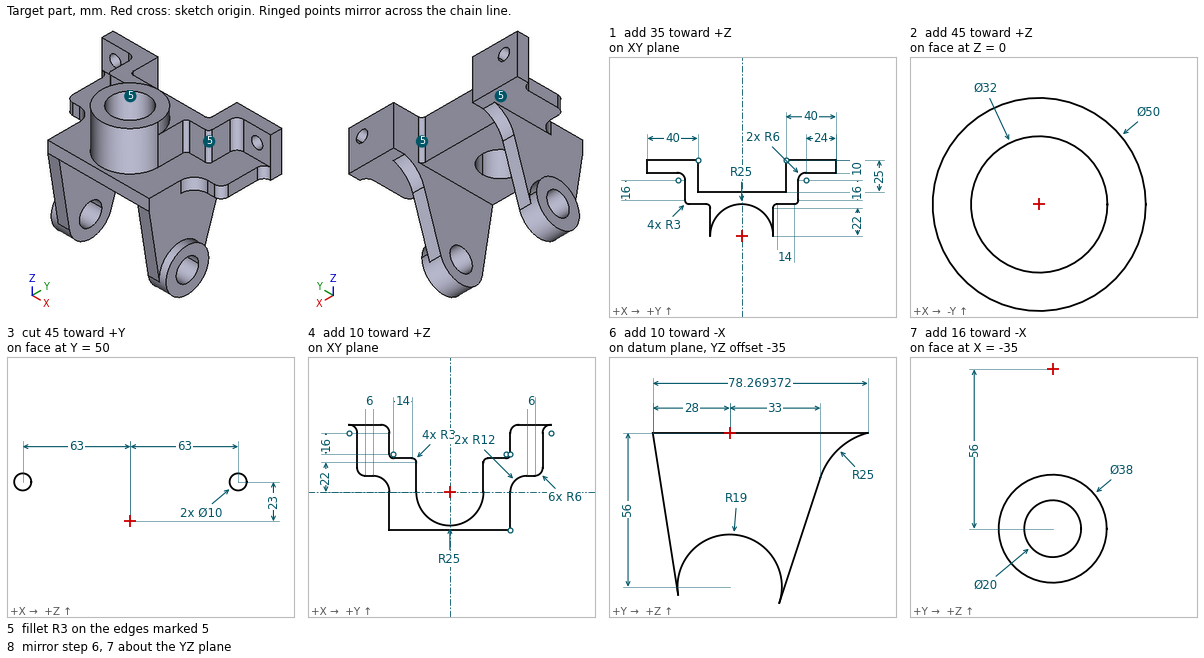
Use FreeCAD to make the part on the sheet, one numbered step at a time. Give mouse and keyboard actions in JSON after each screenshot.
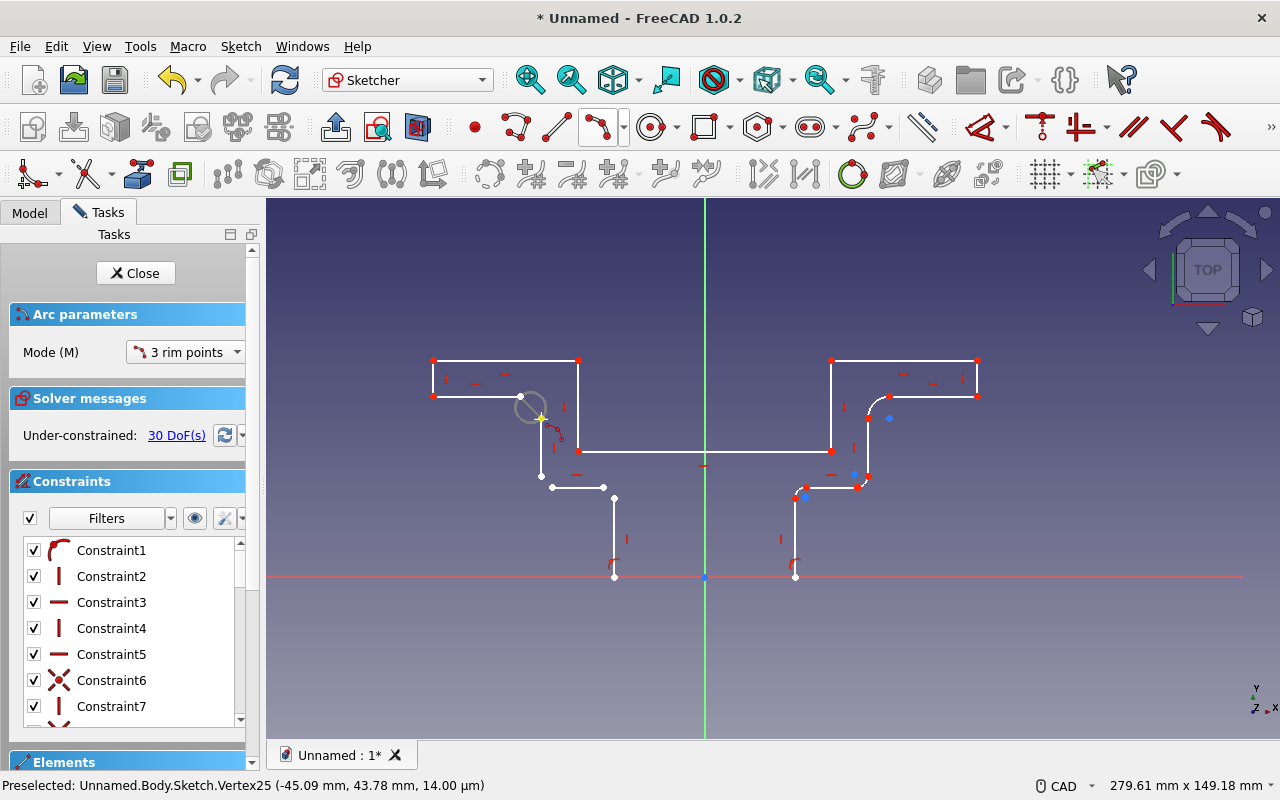
{"action": "scroll", "coordinate": [535, 402], "scroll_direction": "up", "scroll_amount": 5}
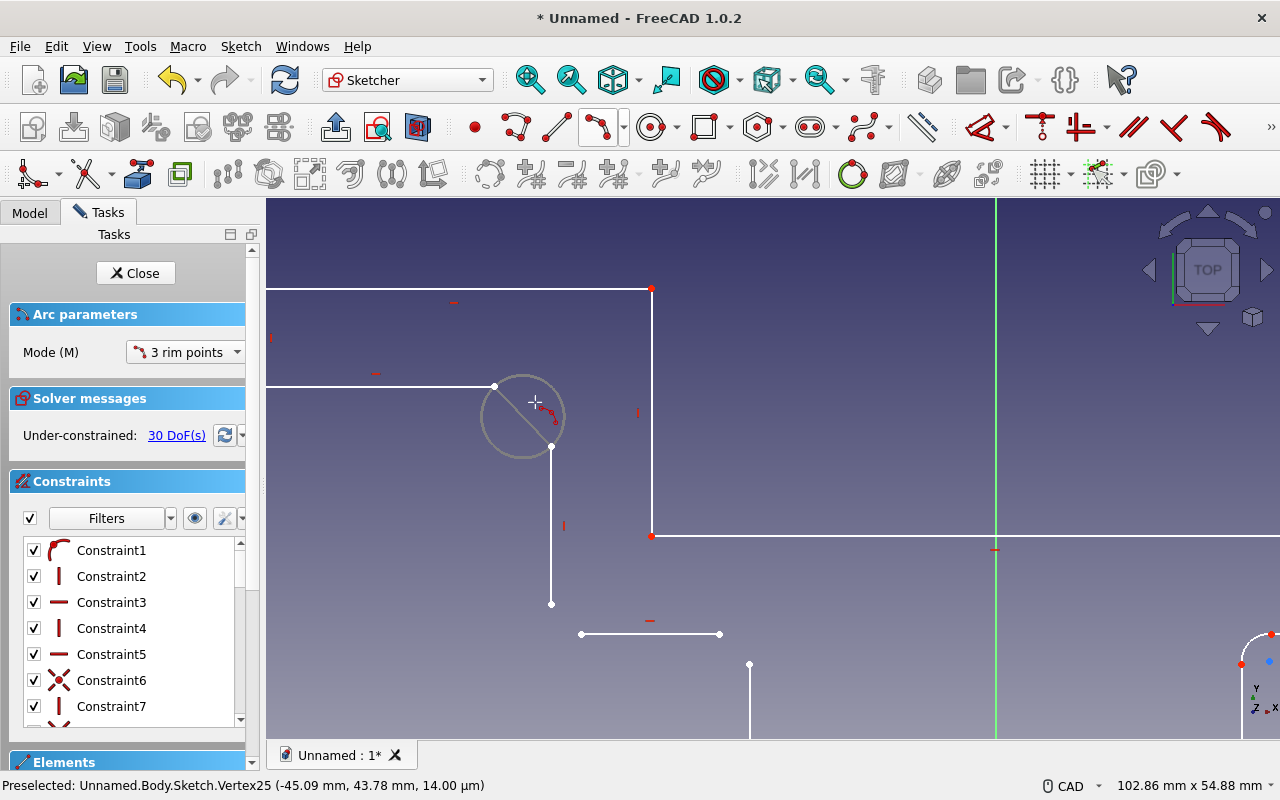
{"action": "left_click", "coordinate": [535, 403]}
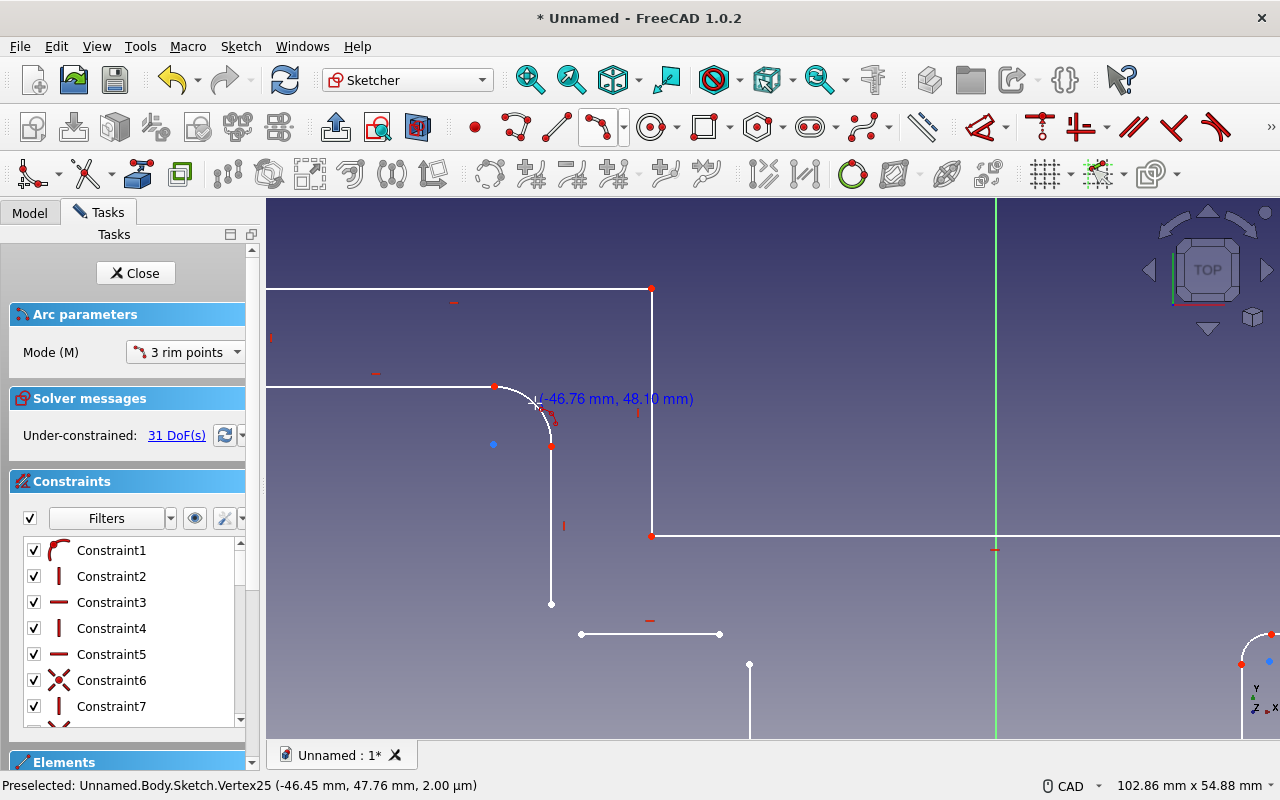
{"action": "left_click", "coordinate": [551, 604]}
{"action": "left_click", "coordinate": [581, 634]}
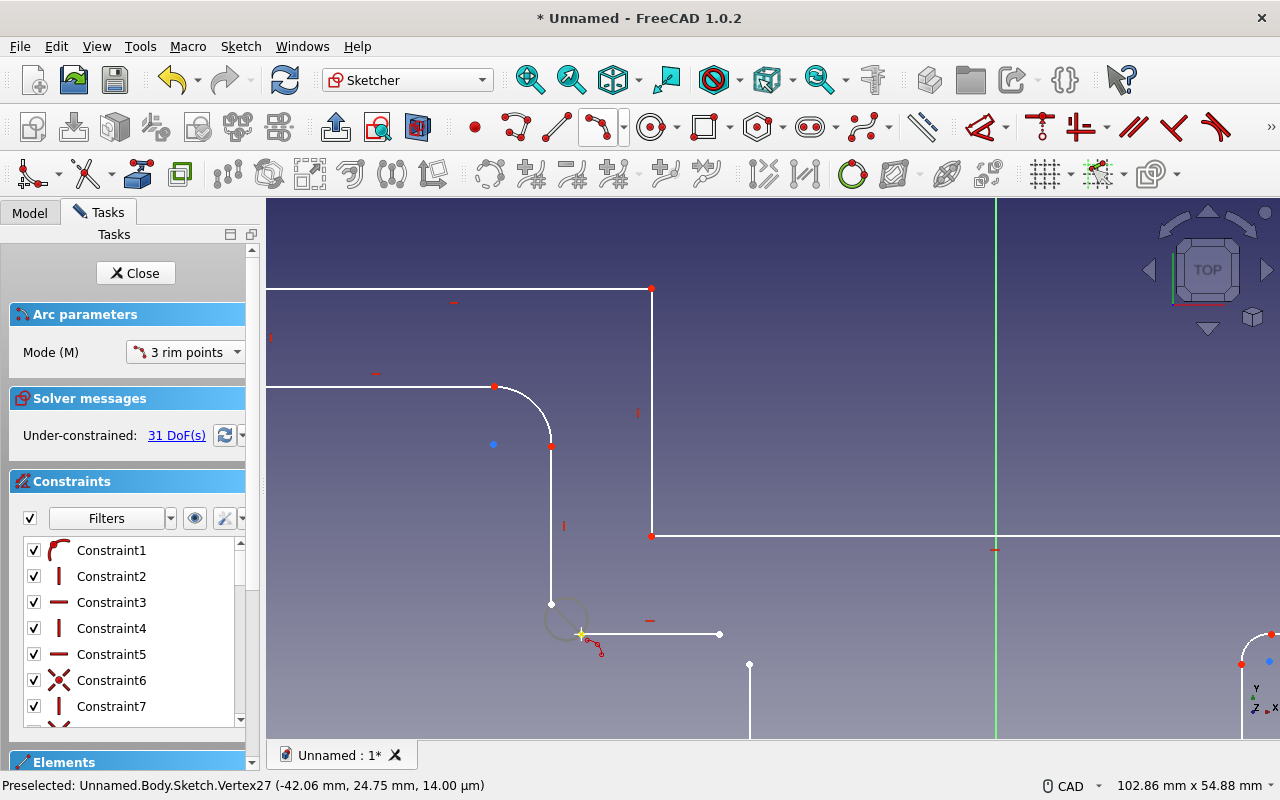
{"action": "scroll", "coordinate": [561, 623], "scroll_direction": "up", "scroll_amount": 4}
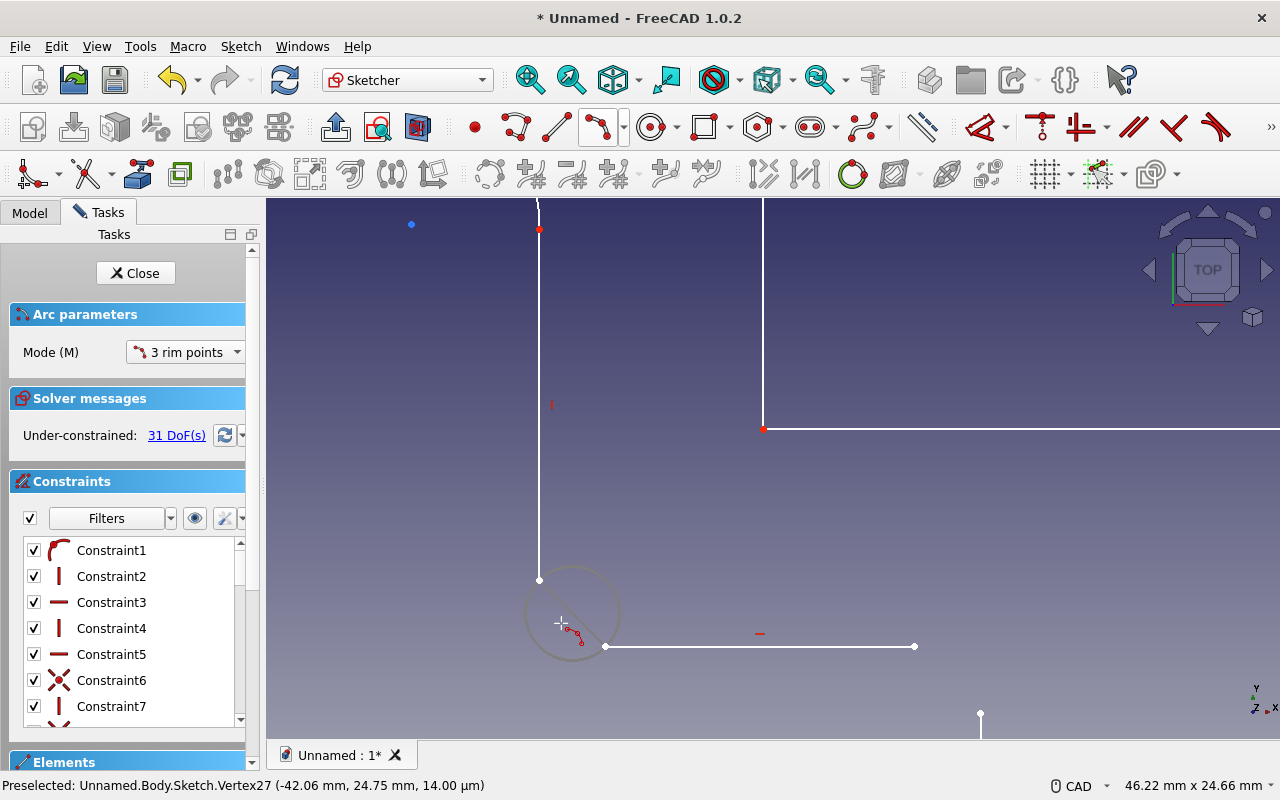
{"action": "left_click", "coordinate": [561, 622]}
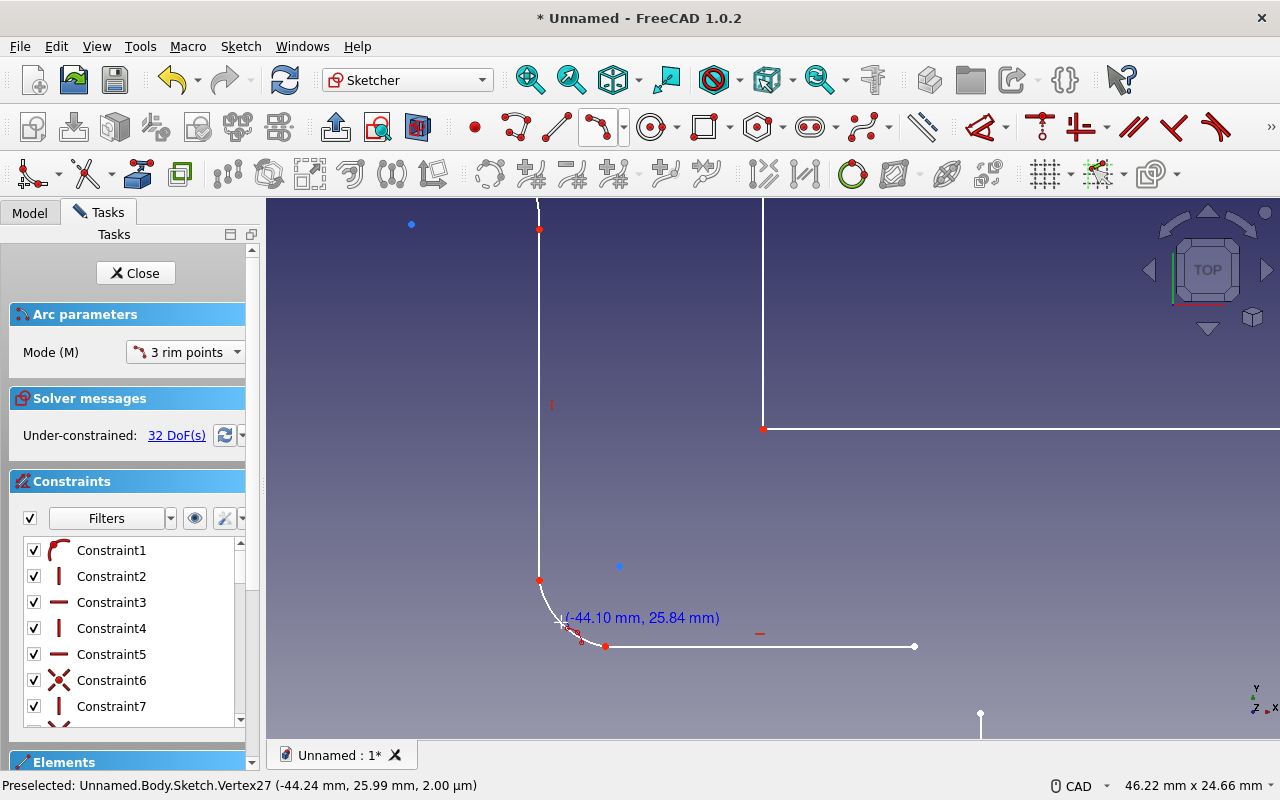
{"action": "scroll", "coordinate": [541, 456], "scroll_direction": "down", "scroll_amount": 9}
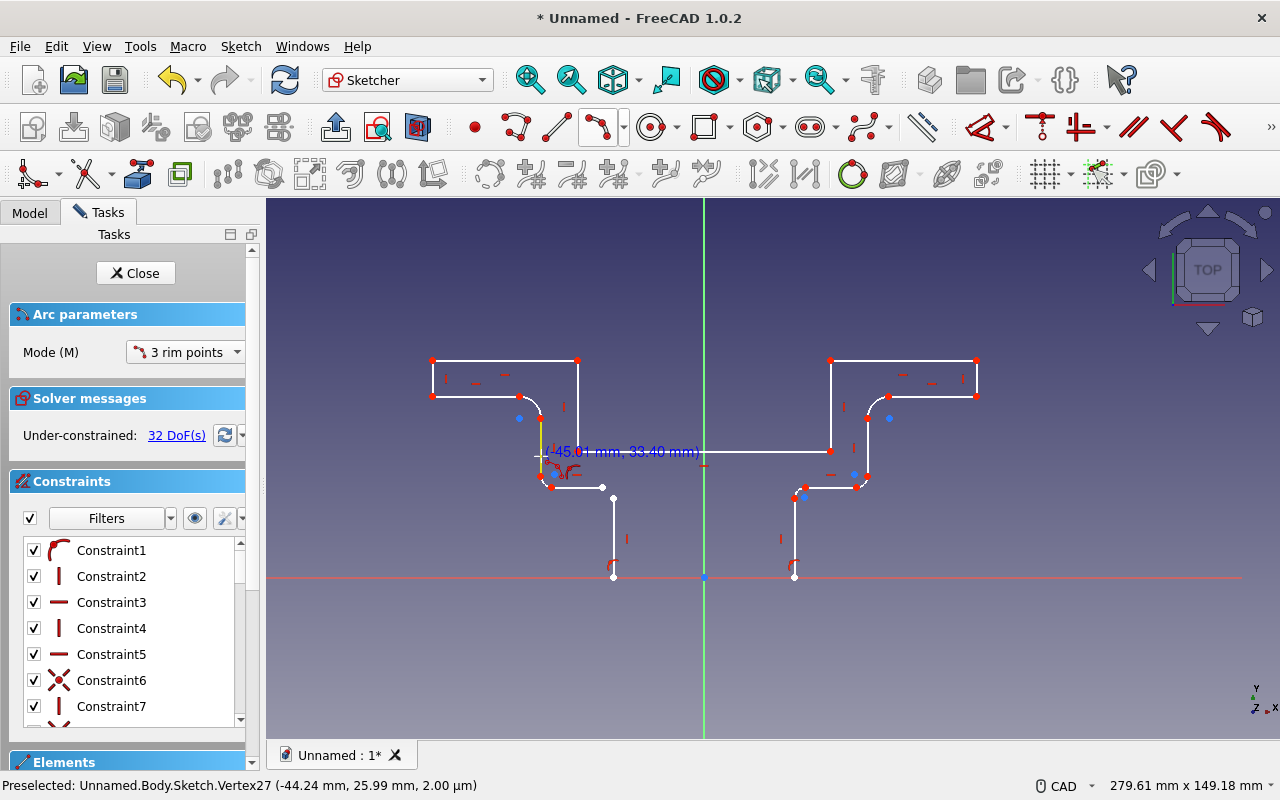
{"action": "left_click", "coordinate": [603, 488]}
{"action": "left_click", "coordinate": [614, 499]}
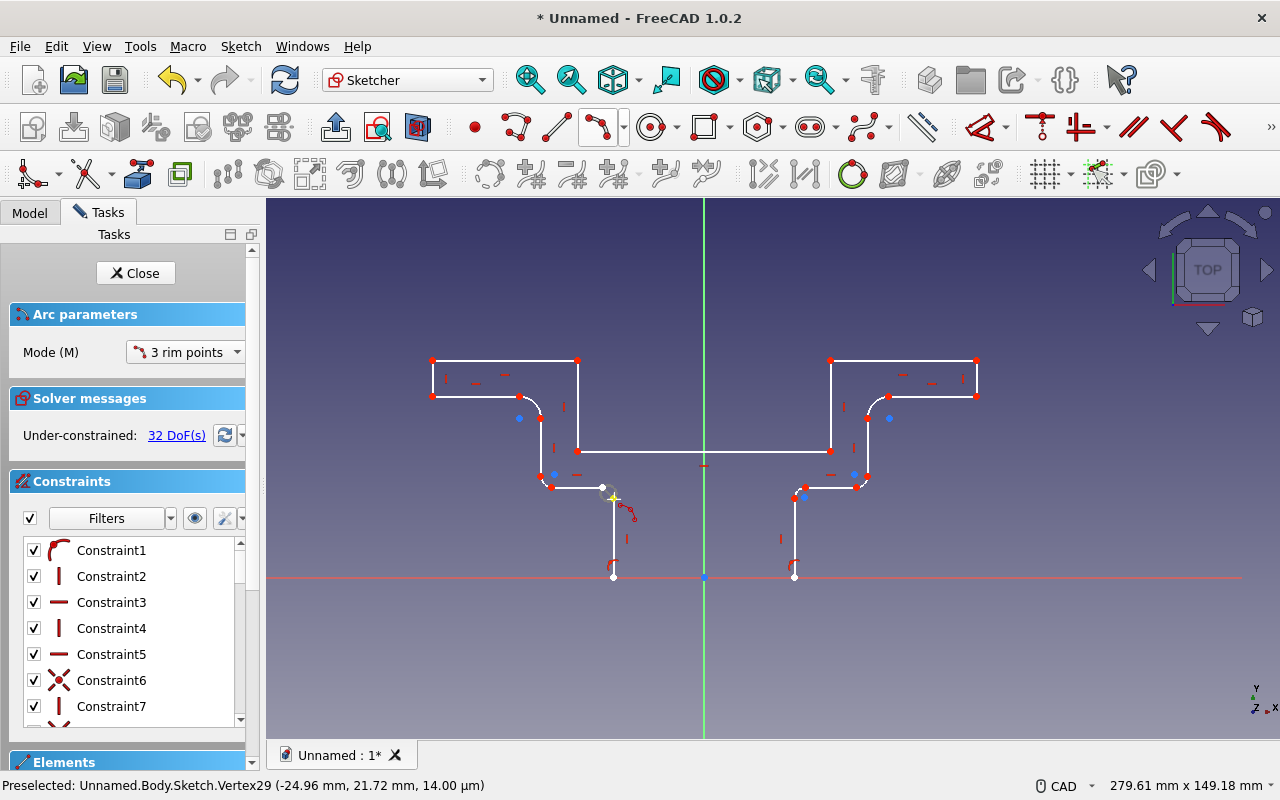
{"action": "scroll", "coordinate": [611, 490], "scroll_direction": "up", "scroll_amount": 9}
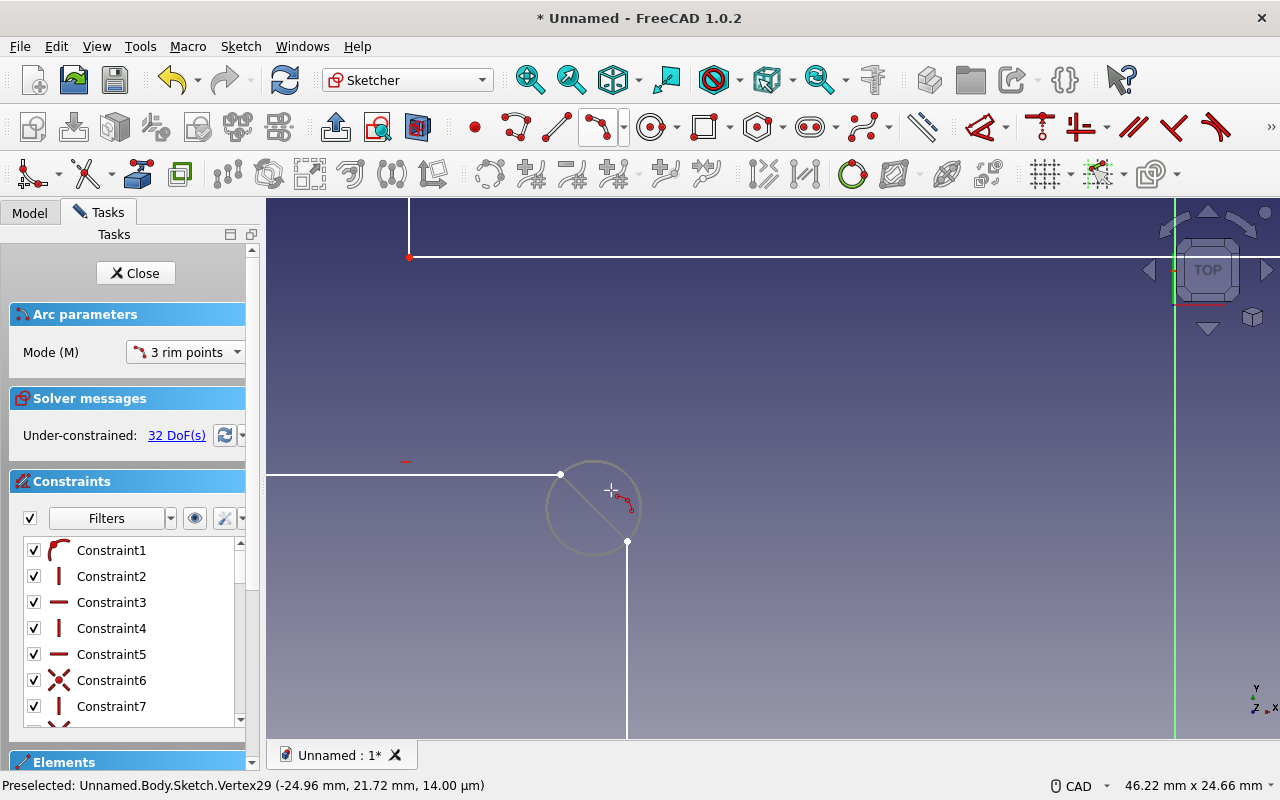
{"action": "left_click", "coordinate": [607, 489]}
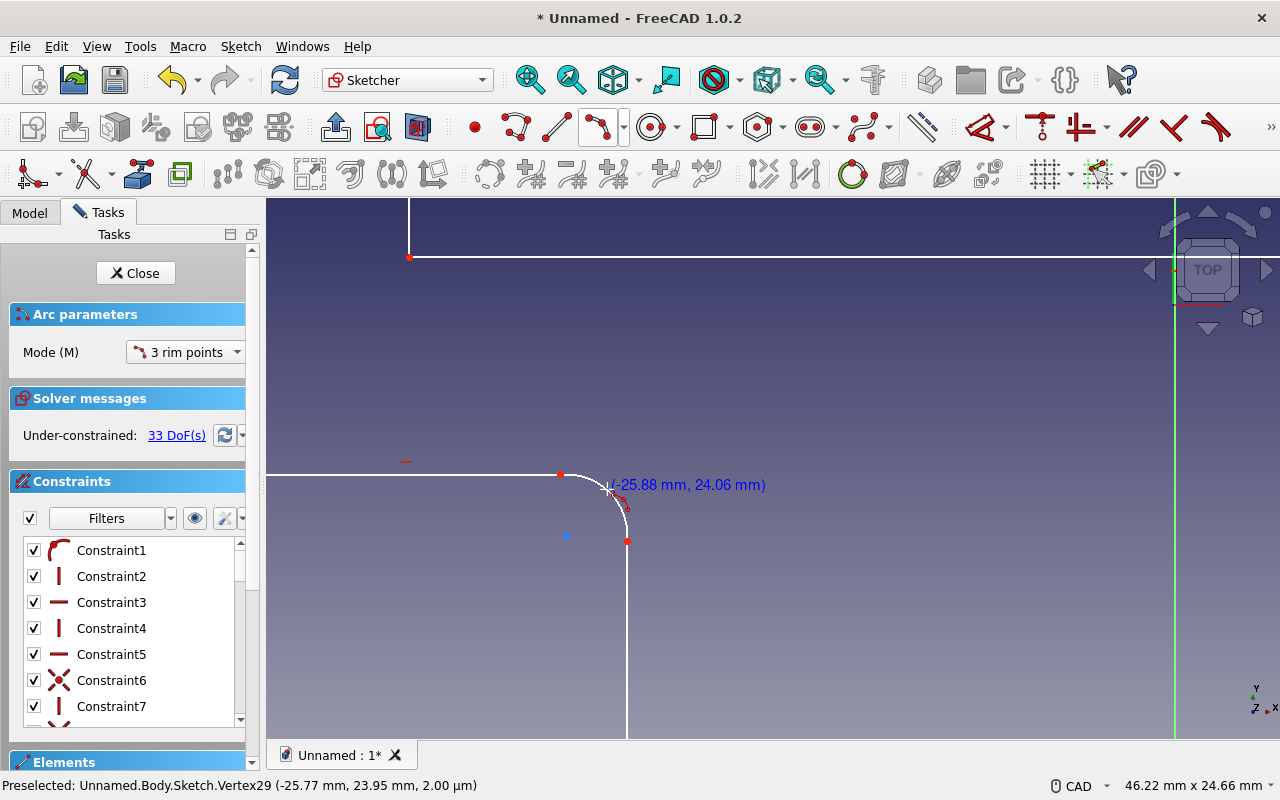
{"action": "scroll", "coordinate": [611, 490], "scroll_direction": "down", "scroll_amount": 9}